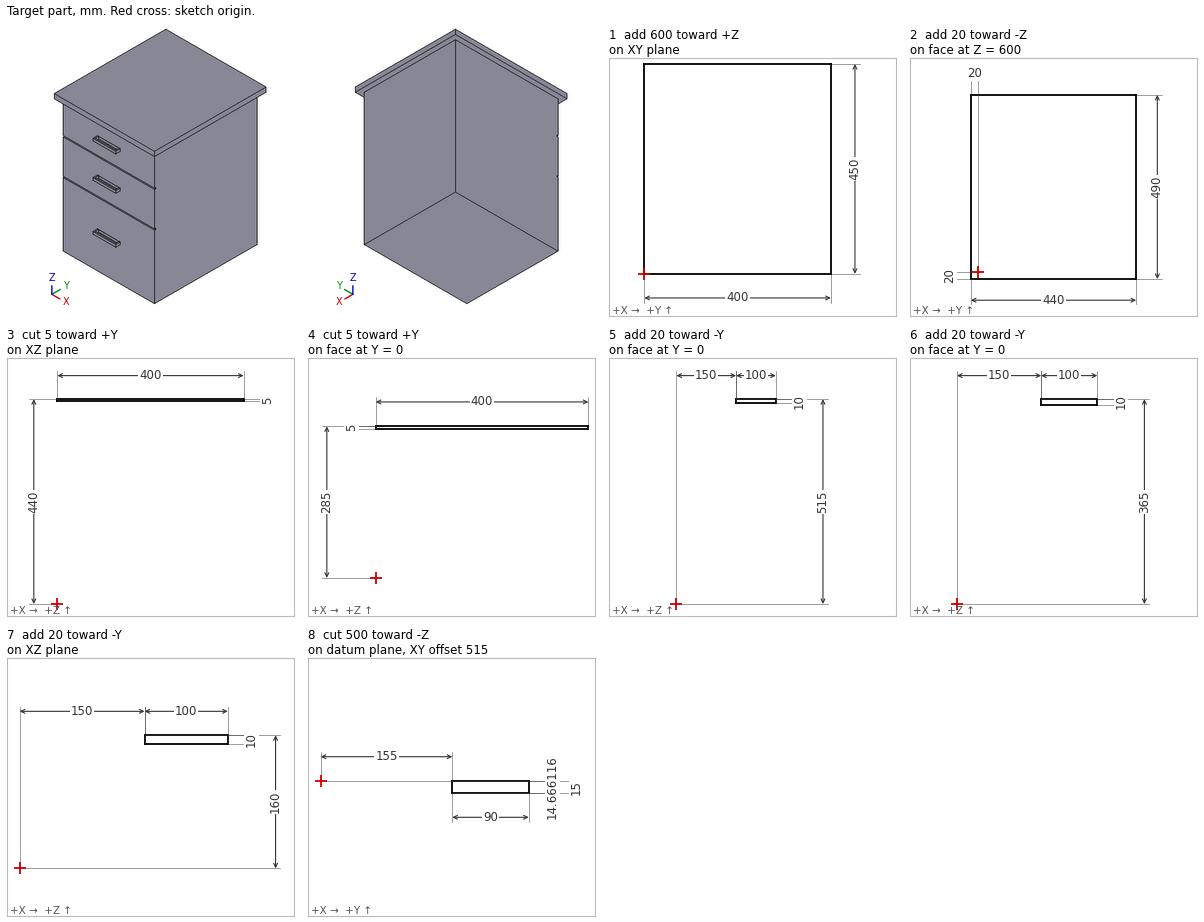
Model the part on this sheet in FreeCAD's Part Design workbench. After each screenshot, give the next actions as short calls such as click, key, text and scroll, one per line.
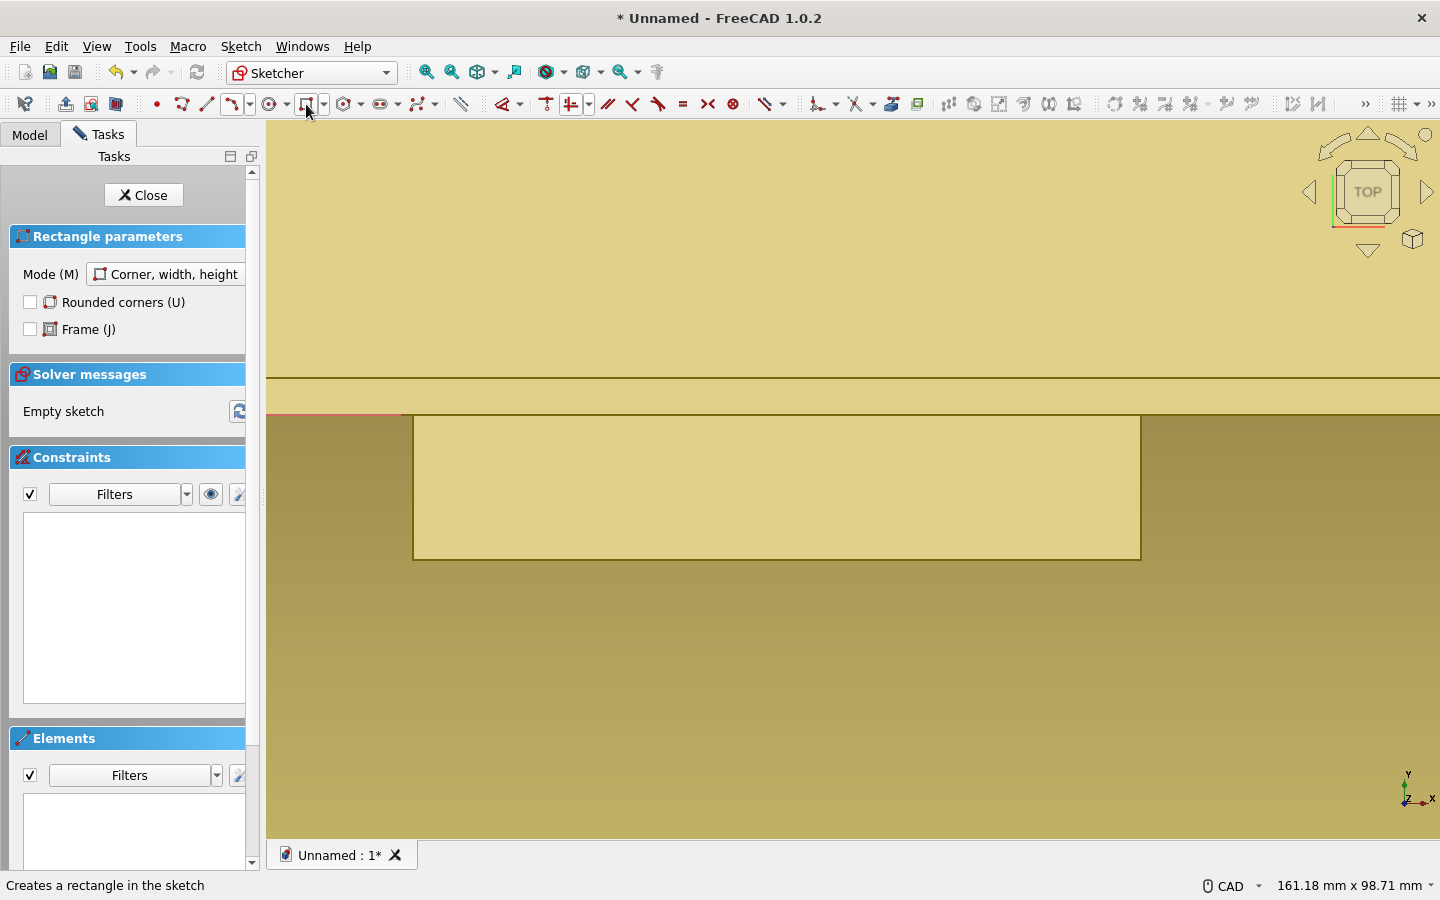
scroll(449, 417, up, 10)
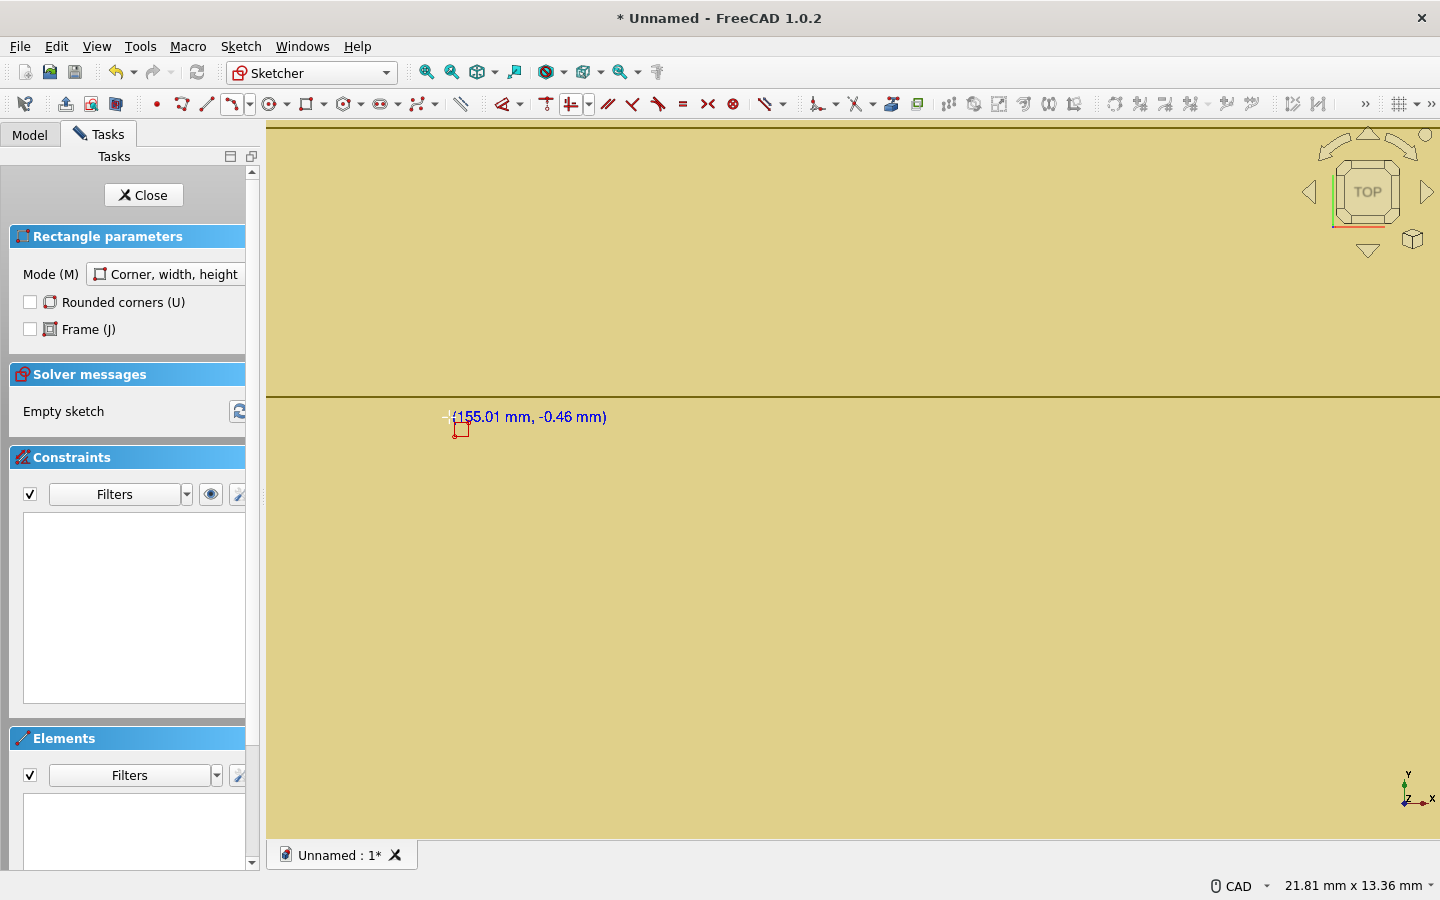
click(448, 415)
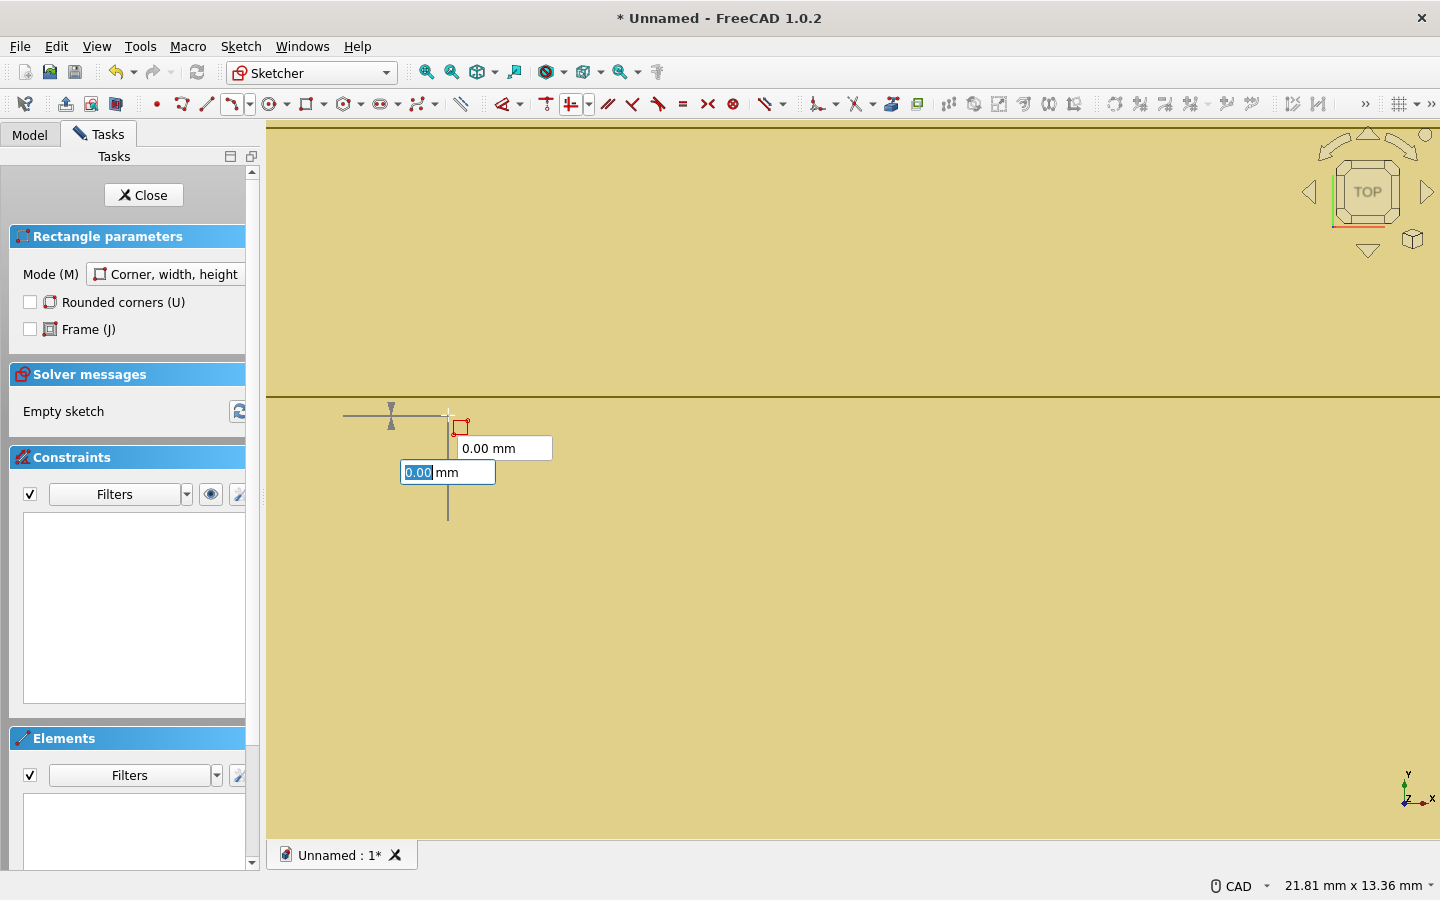
scroll(458, 428, down, 10)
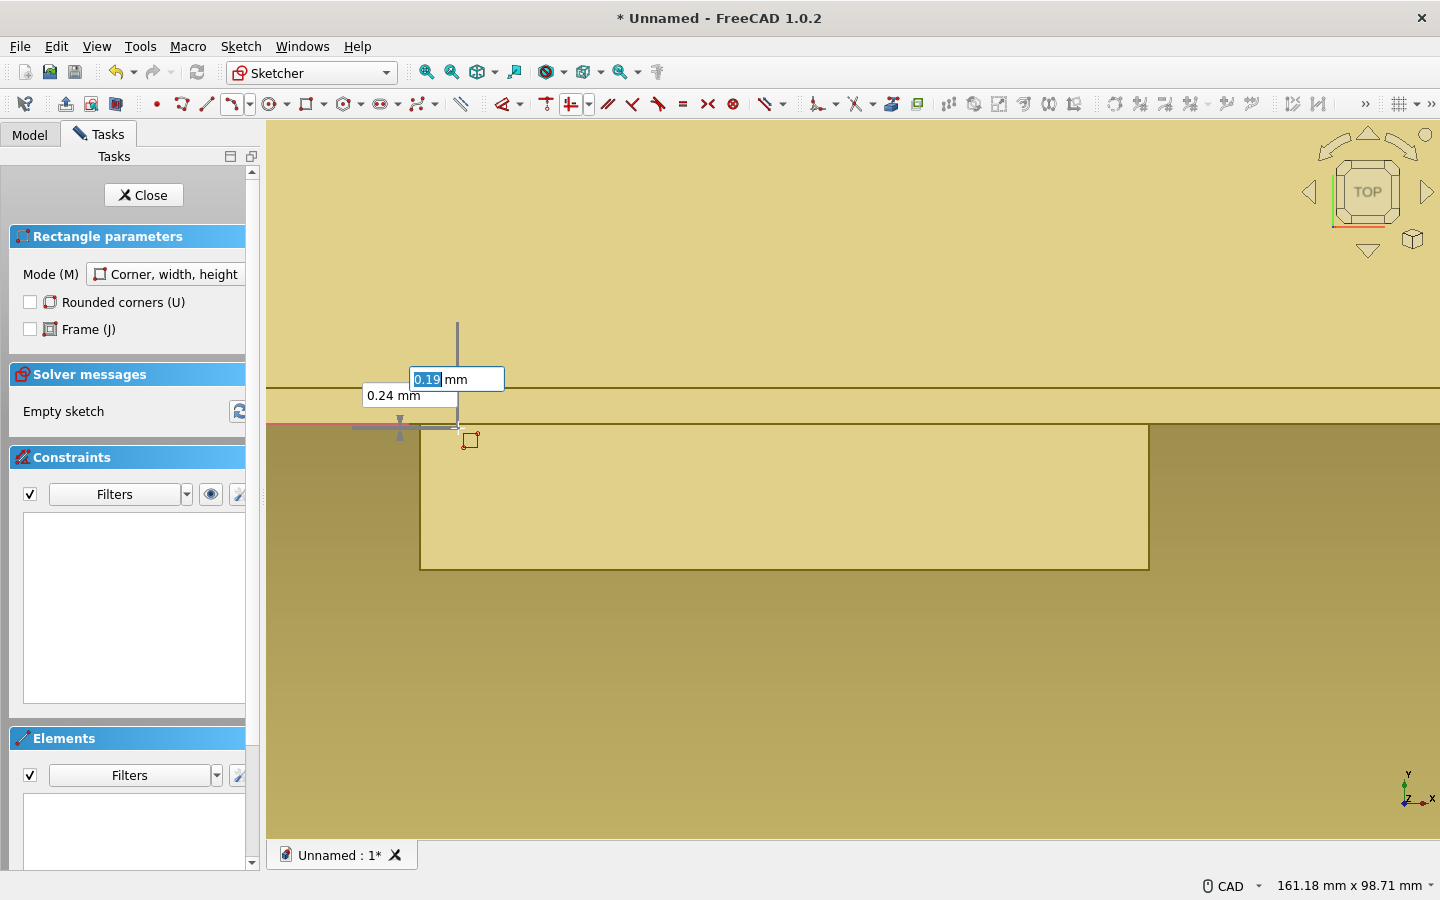
click(1112, 533)
key(Escape)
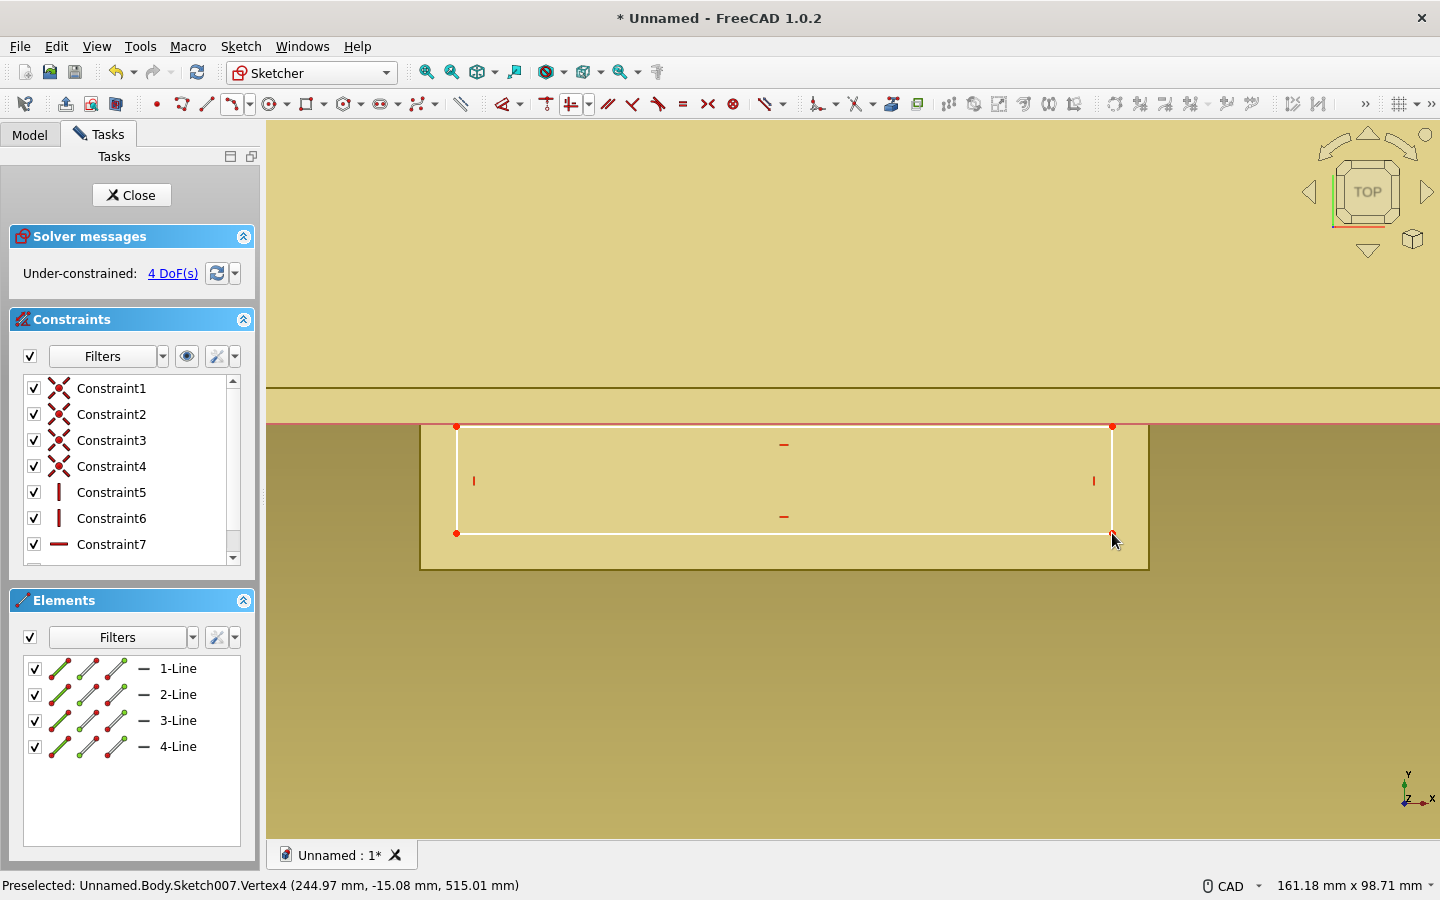
click(502, 104)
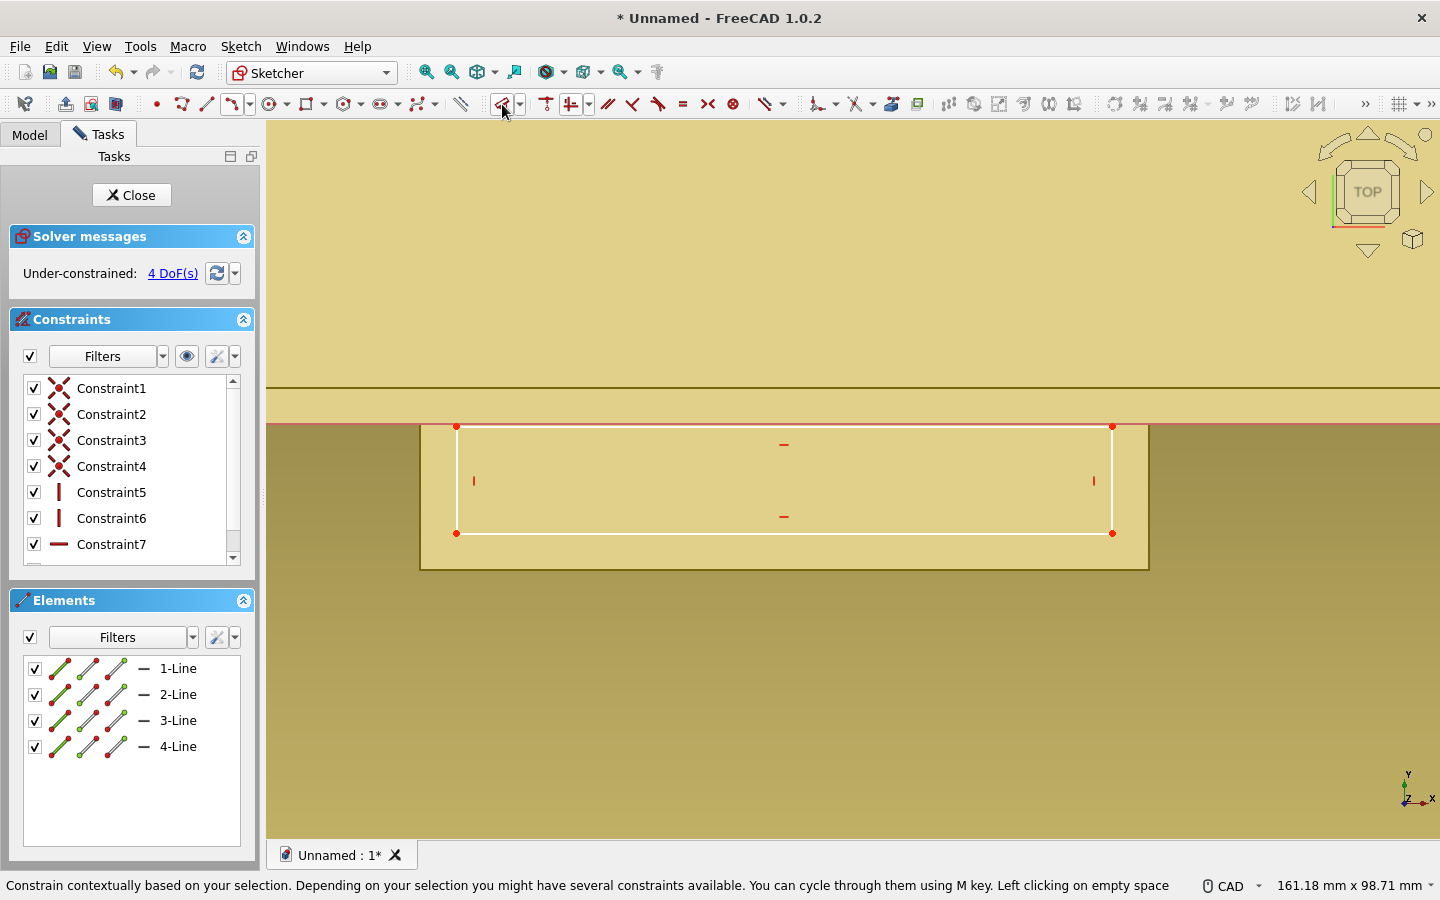
click(653, 534)
click(784, 568)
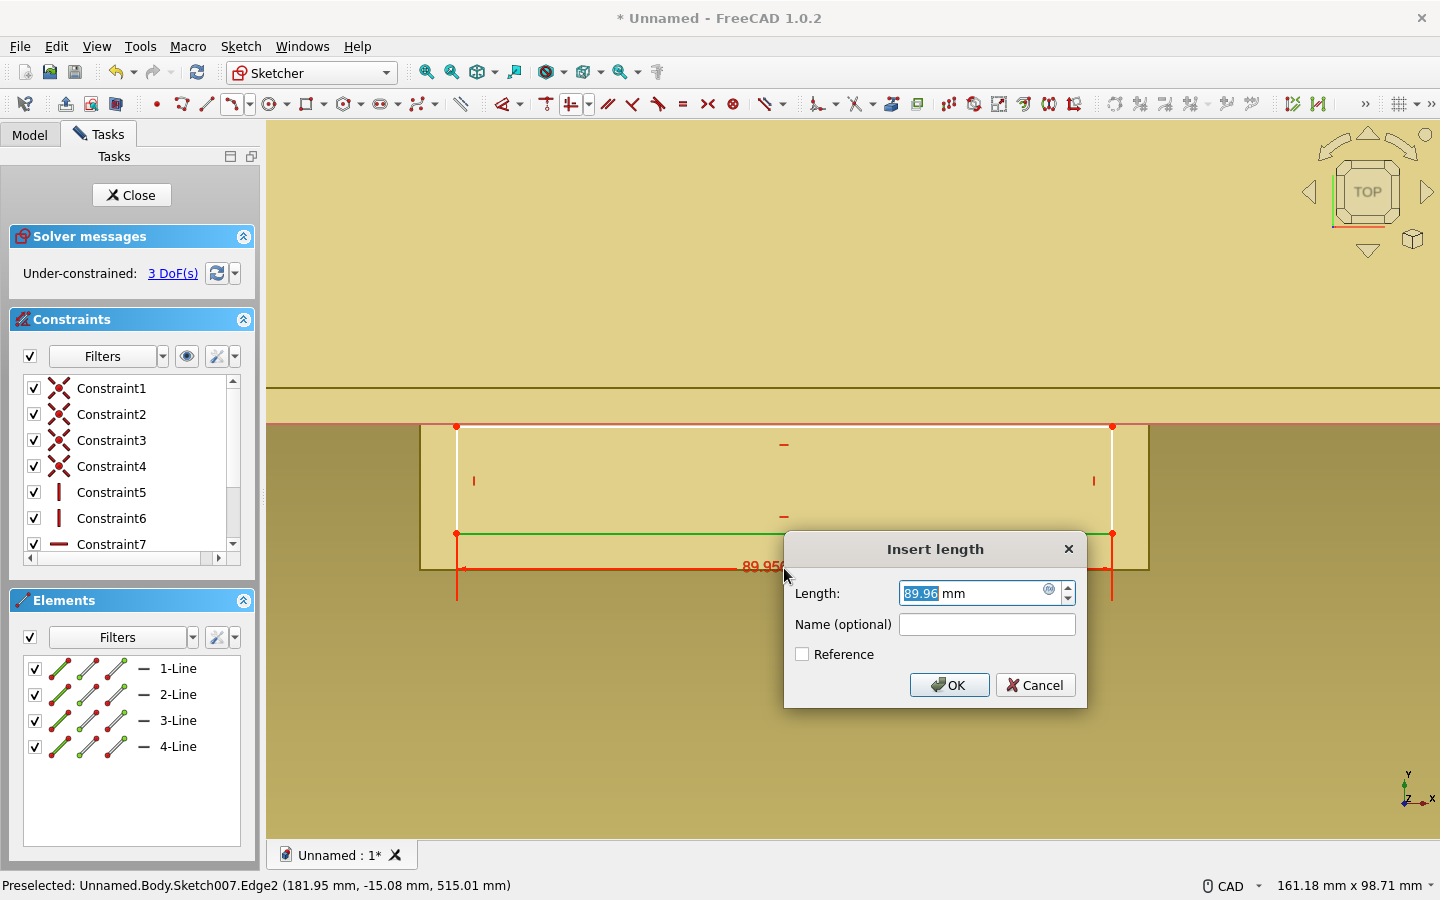
text(90)
key(Return)